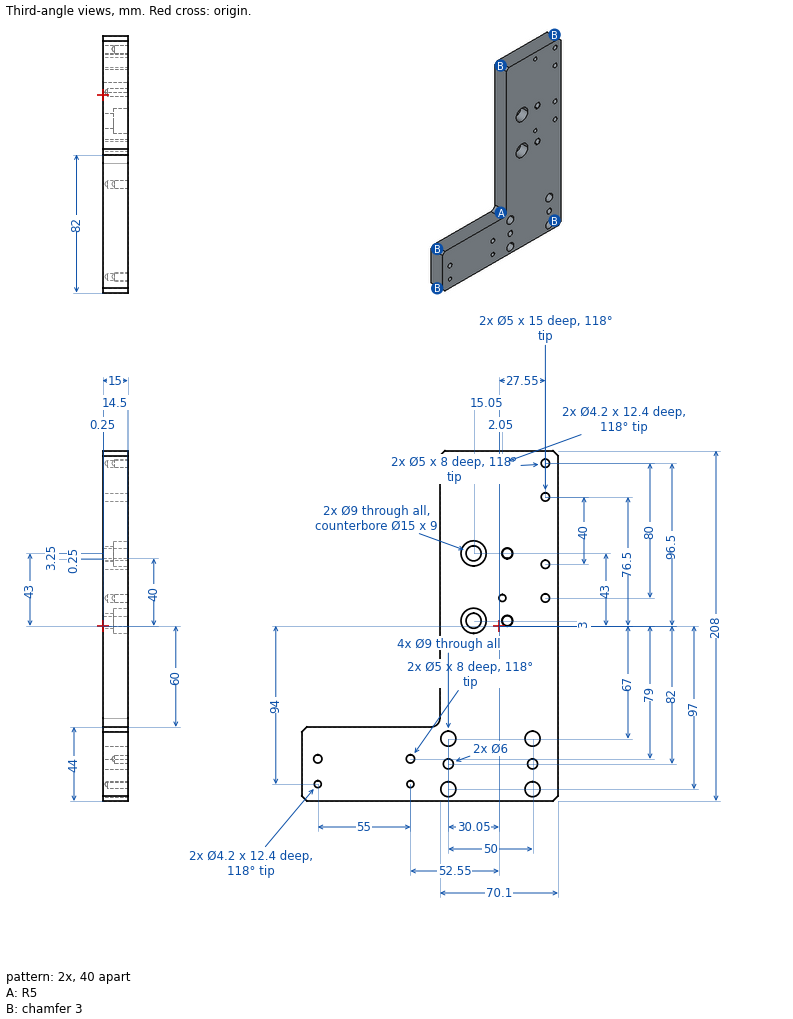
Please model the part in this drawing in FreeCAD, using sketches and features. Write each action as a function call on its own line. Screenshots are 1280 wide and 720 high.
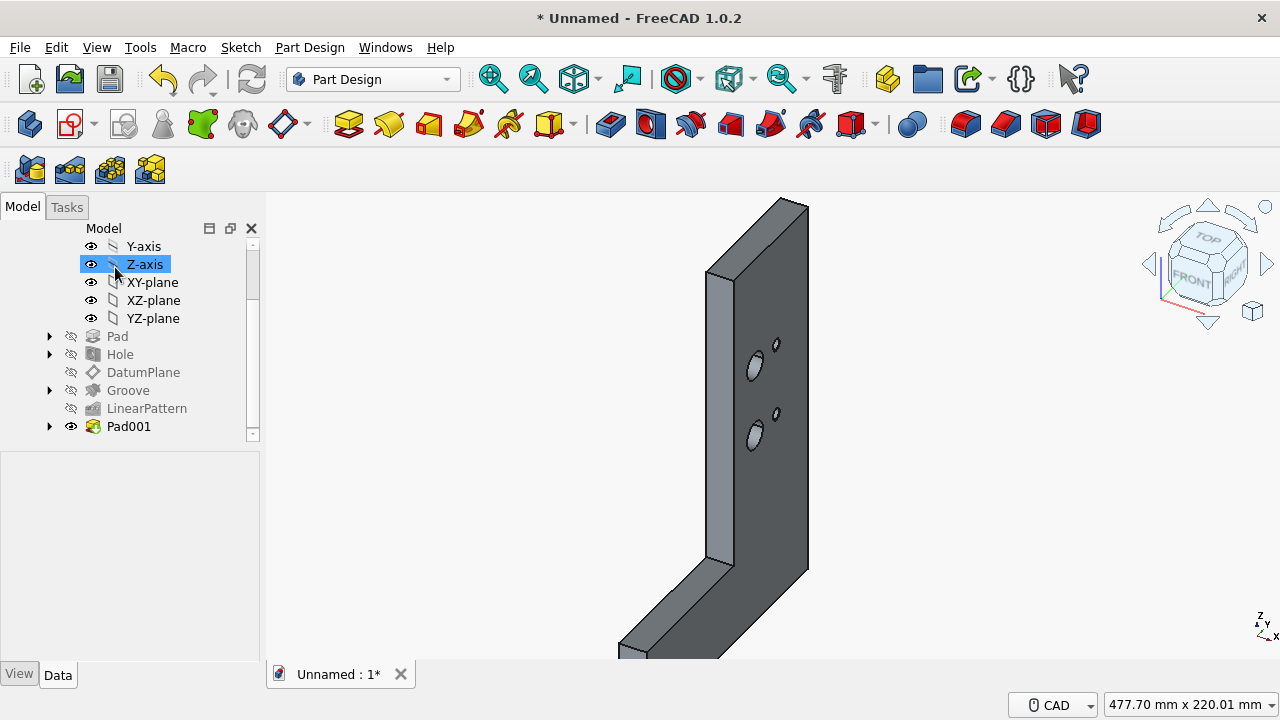
click(494, 80)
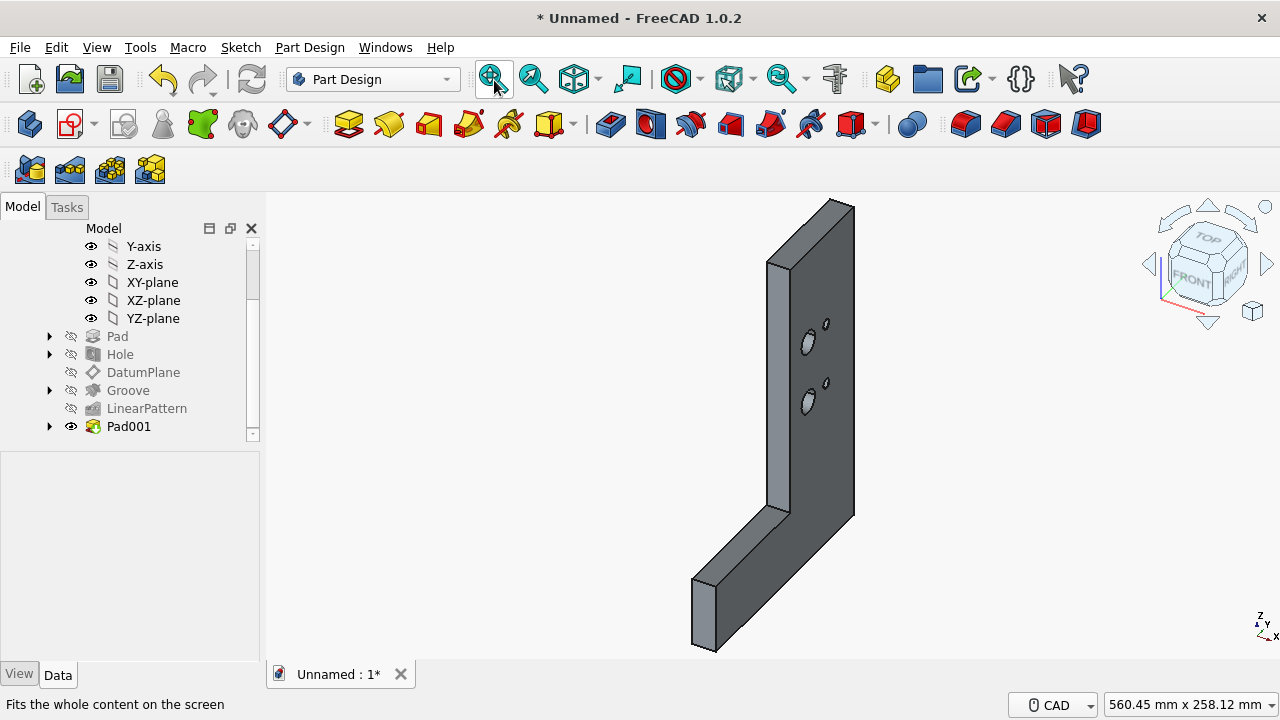
click(824, 477)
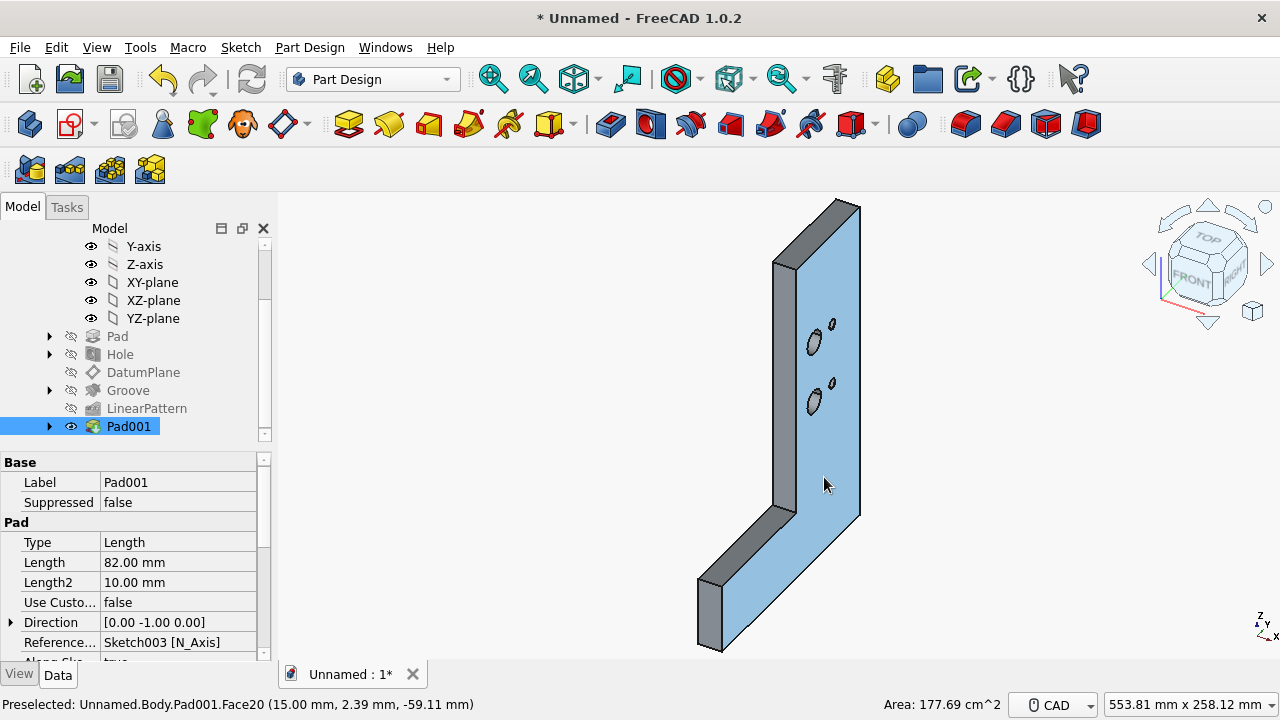
click(70, 124)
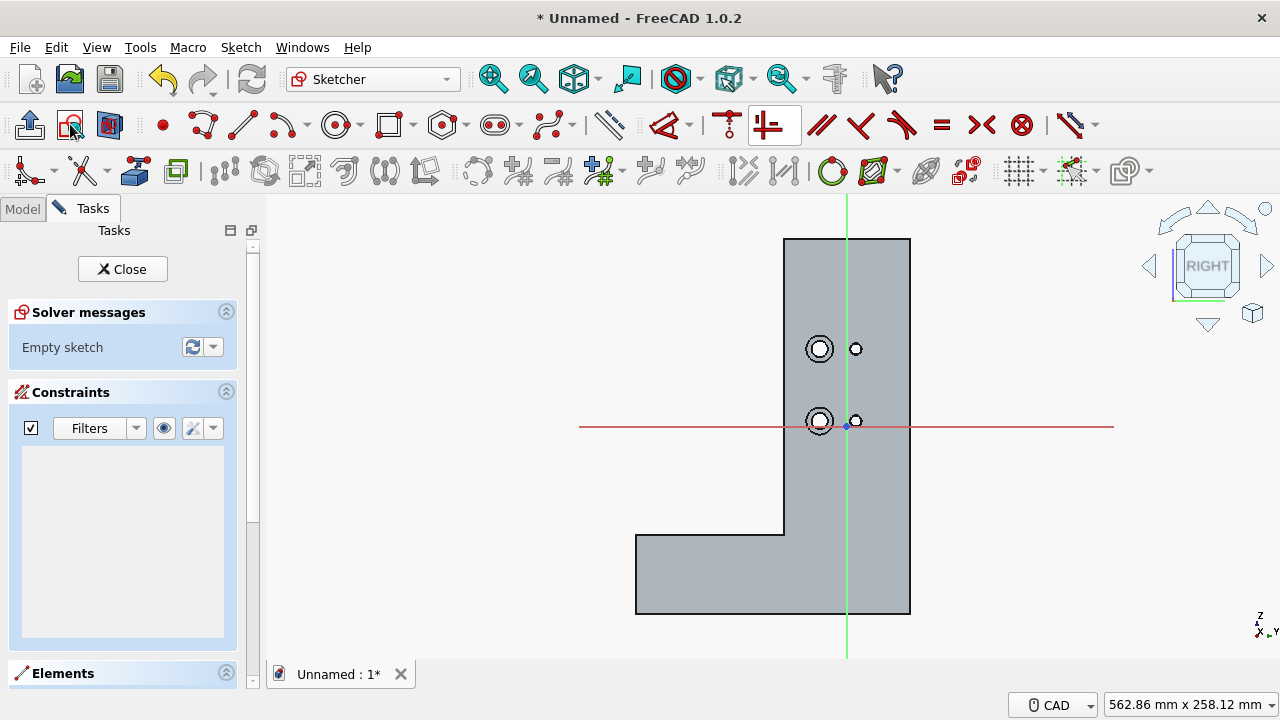
scroll(801, 618, up, 3)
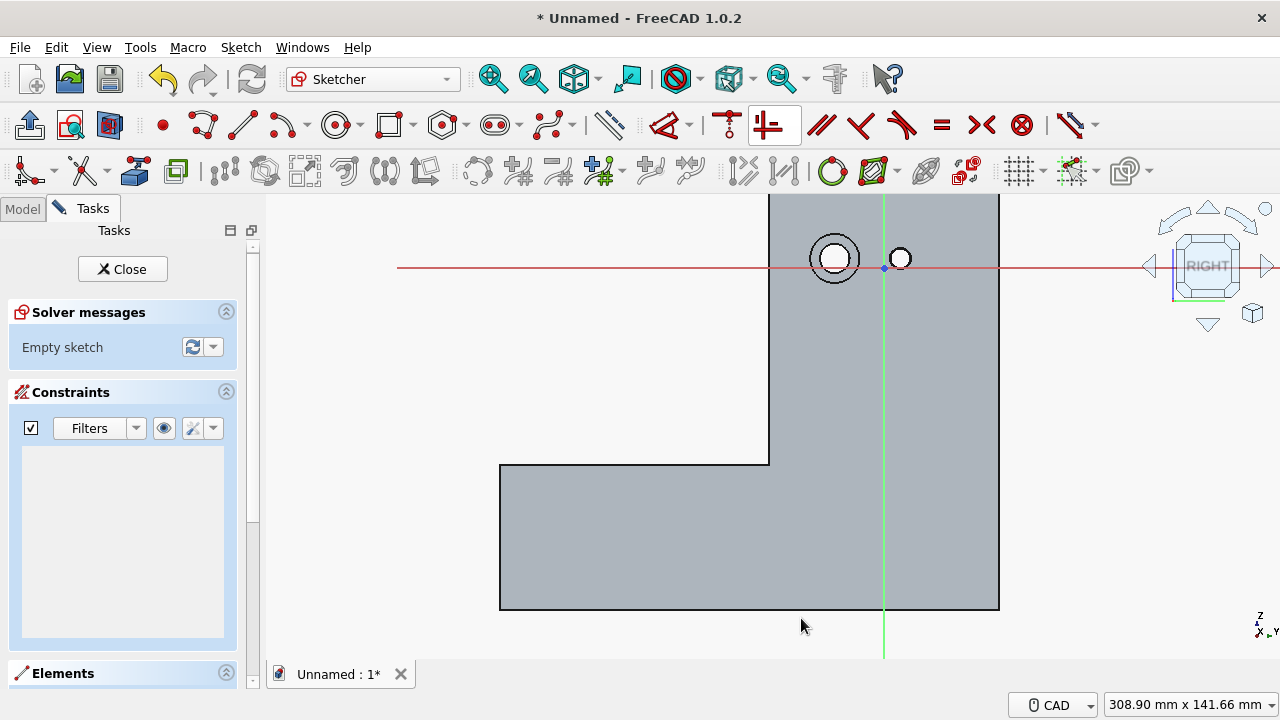
key(g)
key(c)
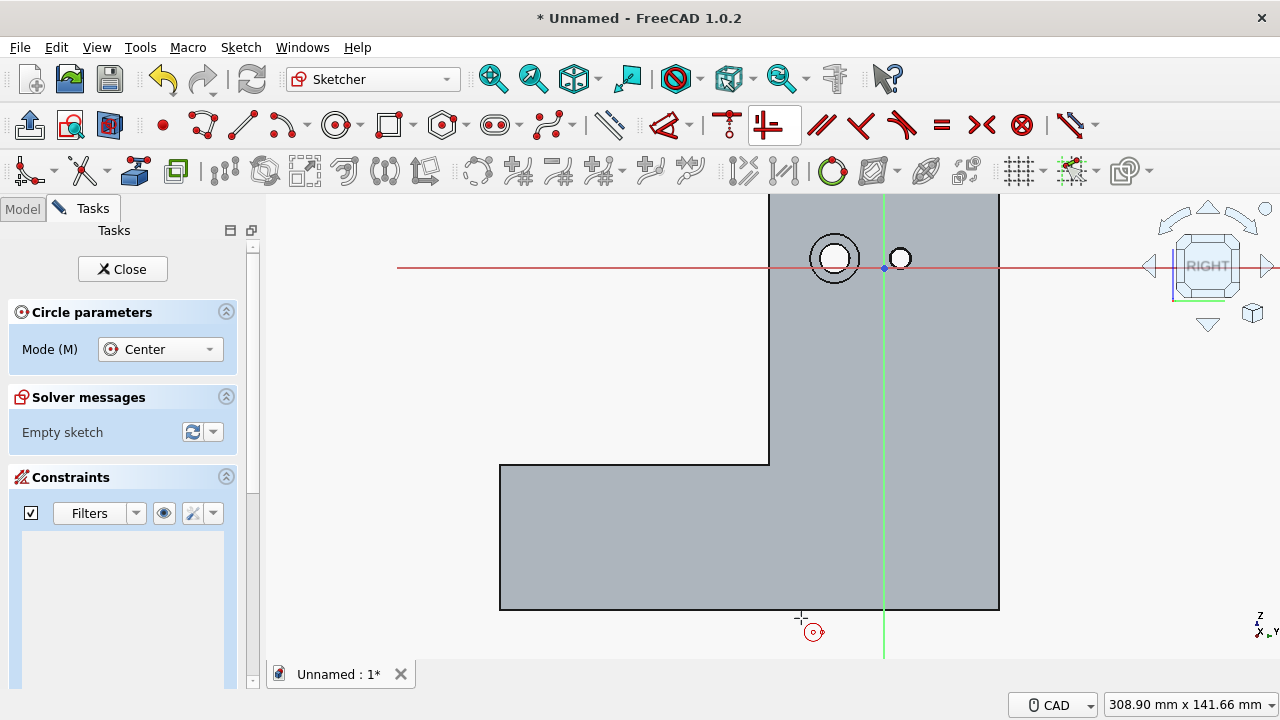
scroll(531, 577, up, 6)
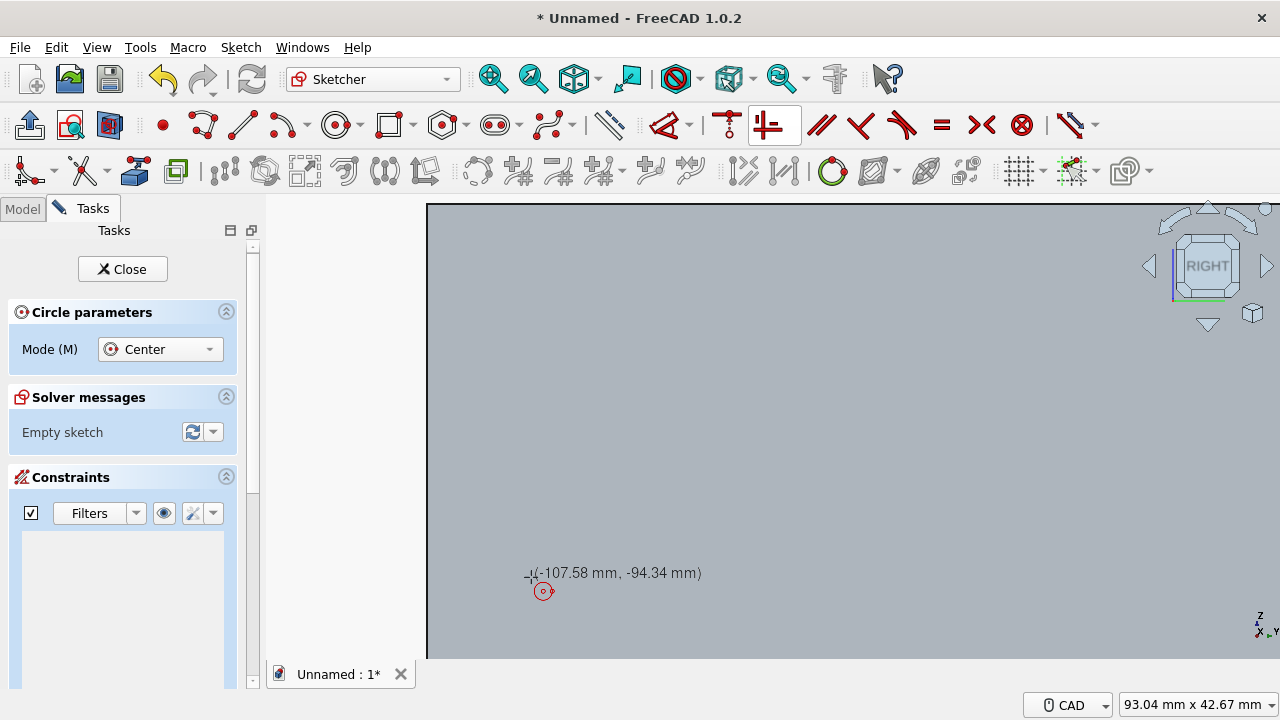
click(531, 575)
click(547, 558)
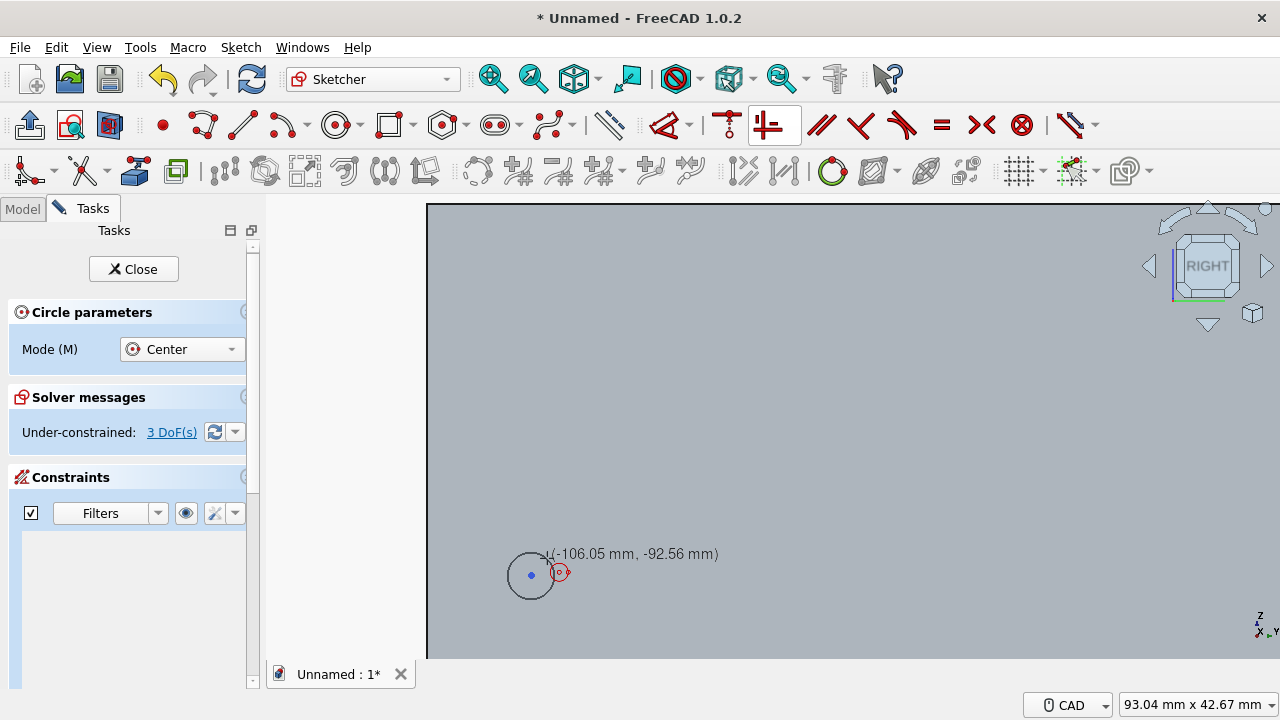
scroll(532, 578, down, 6)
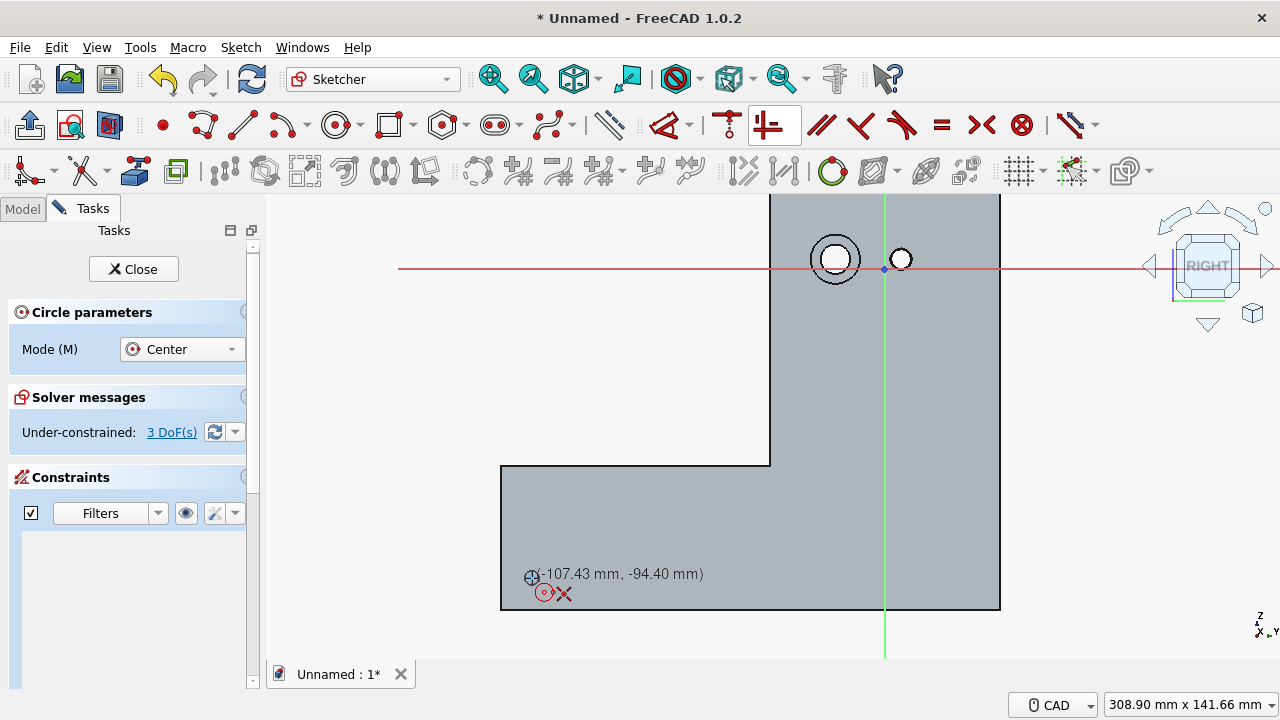
scroll(712, 578, up, 6)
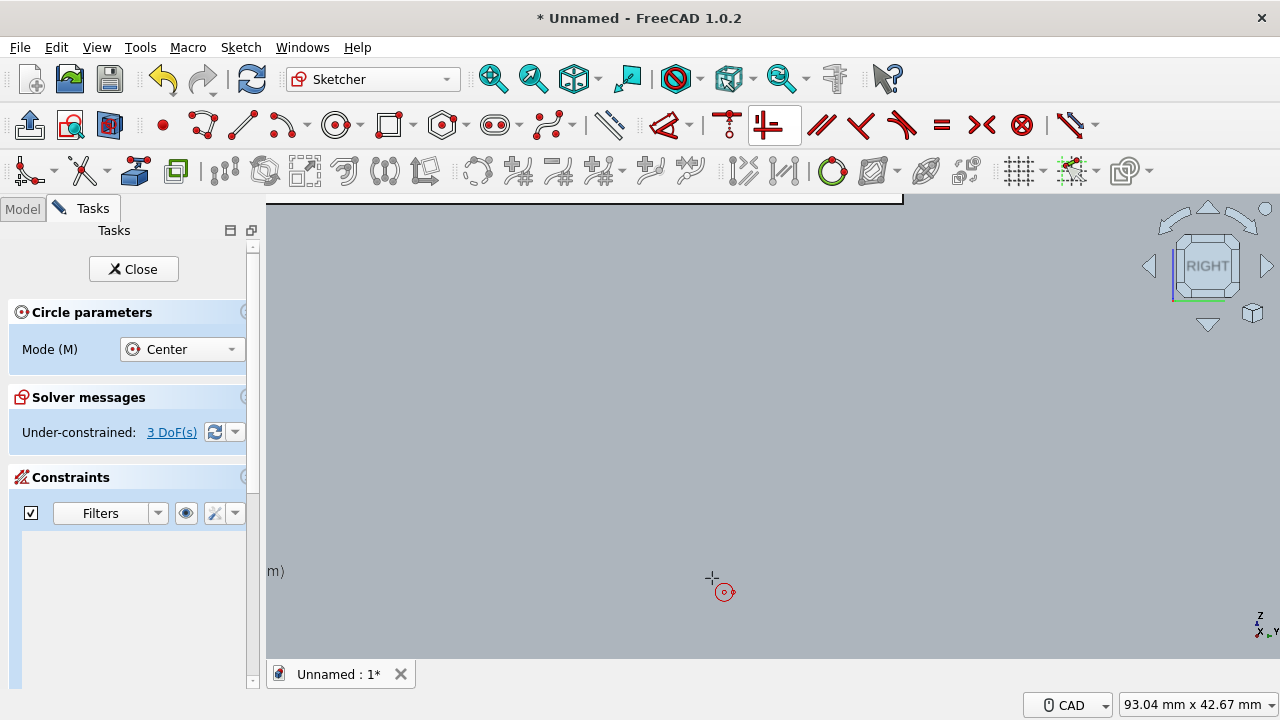
click(712, 575)
click(728, 558)
key(Escape)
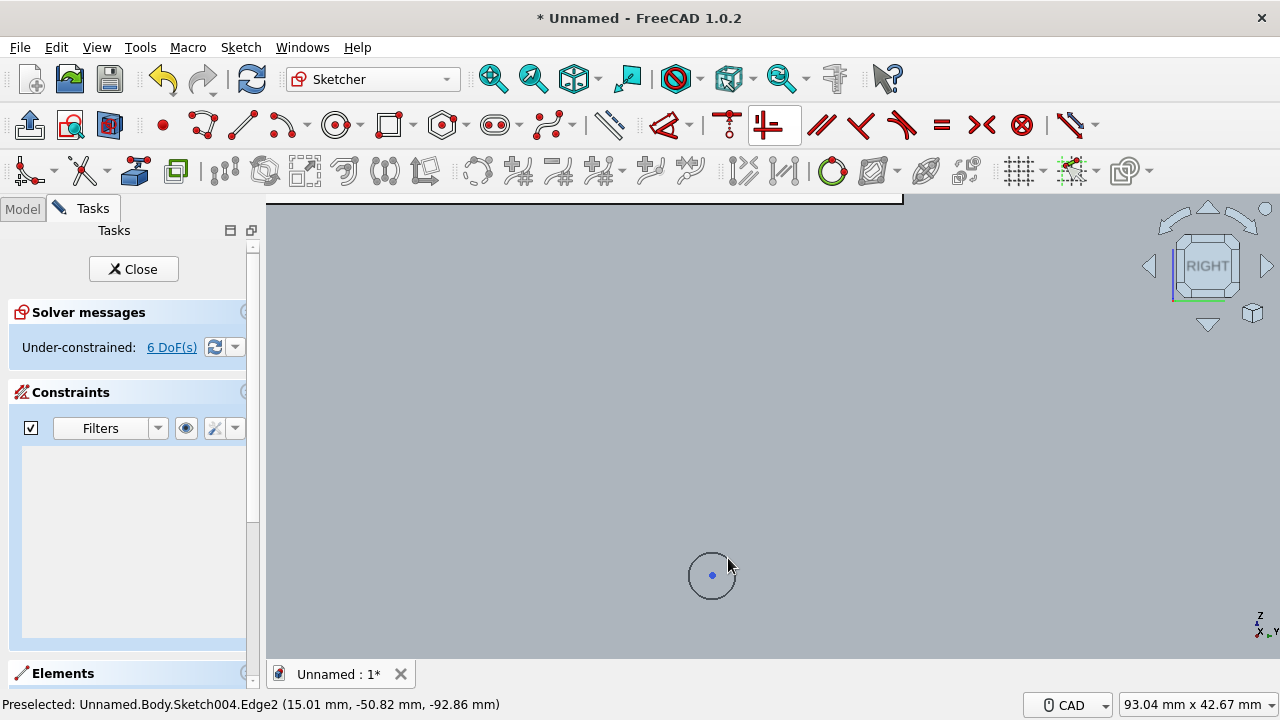
scroll(712, 578, down, 6)